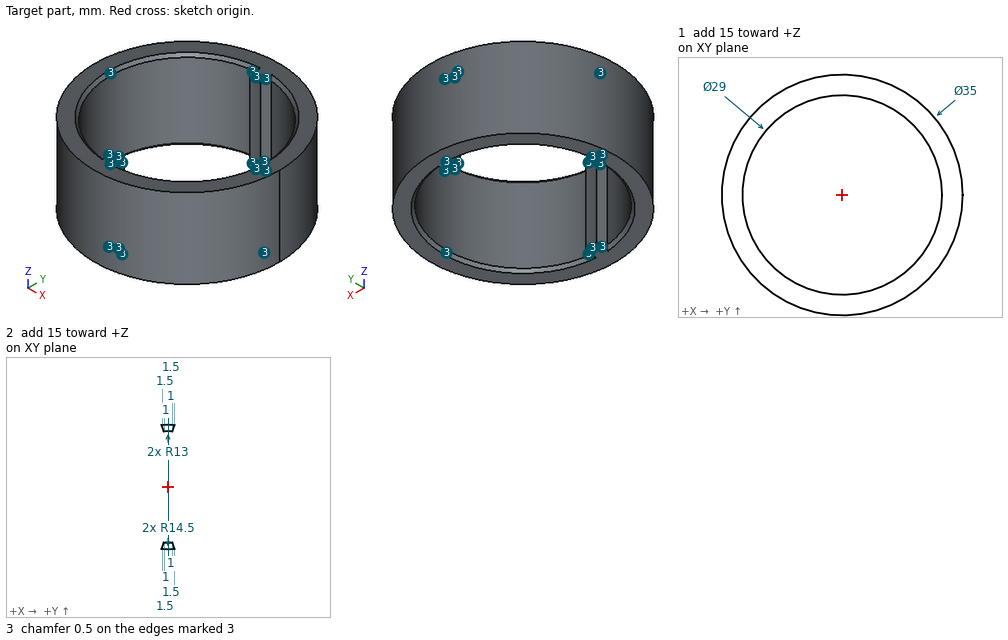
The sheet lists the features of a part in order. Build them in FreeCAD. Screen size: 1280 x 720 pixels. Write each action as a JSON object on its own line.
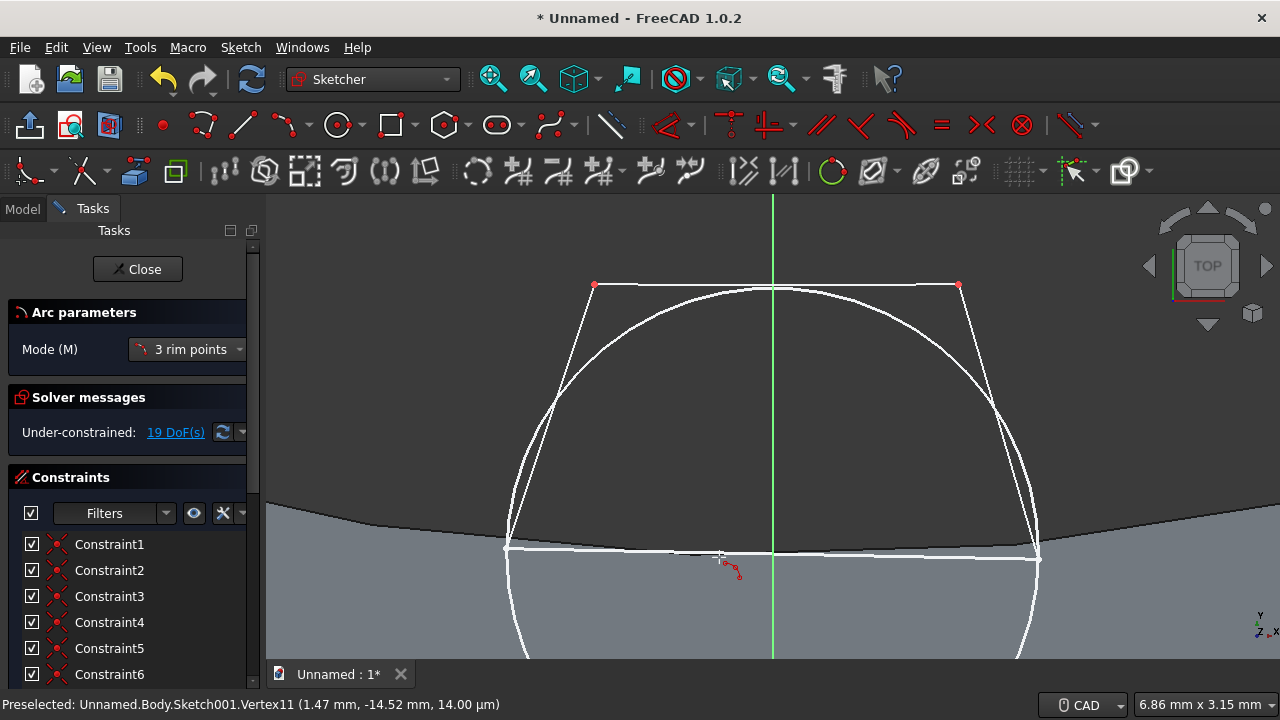
{"action": "left_click", "coordinate": [719, 555]}
{"action": "key", "text": "Escape"}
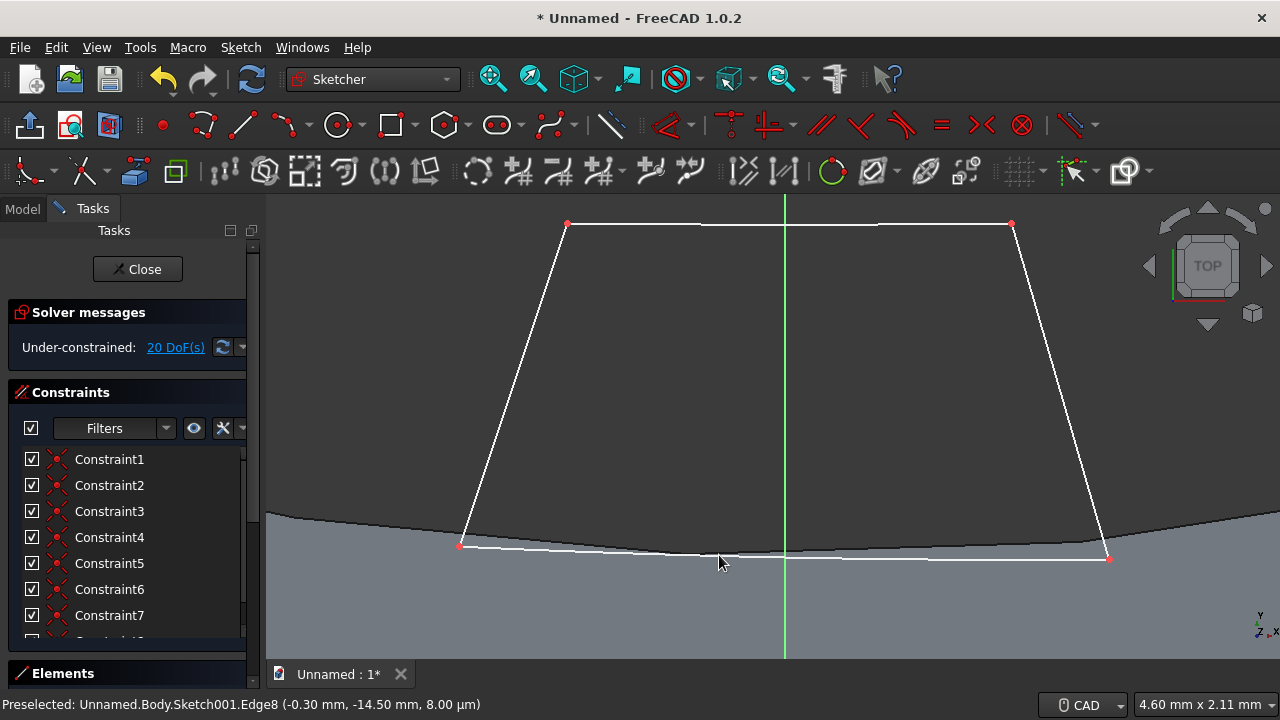
{"action": "scroll", "coordinate": [700, 587], "scroll_direction": "down", "scroll_amount": 15}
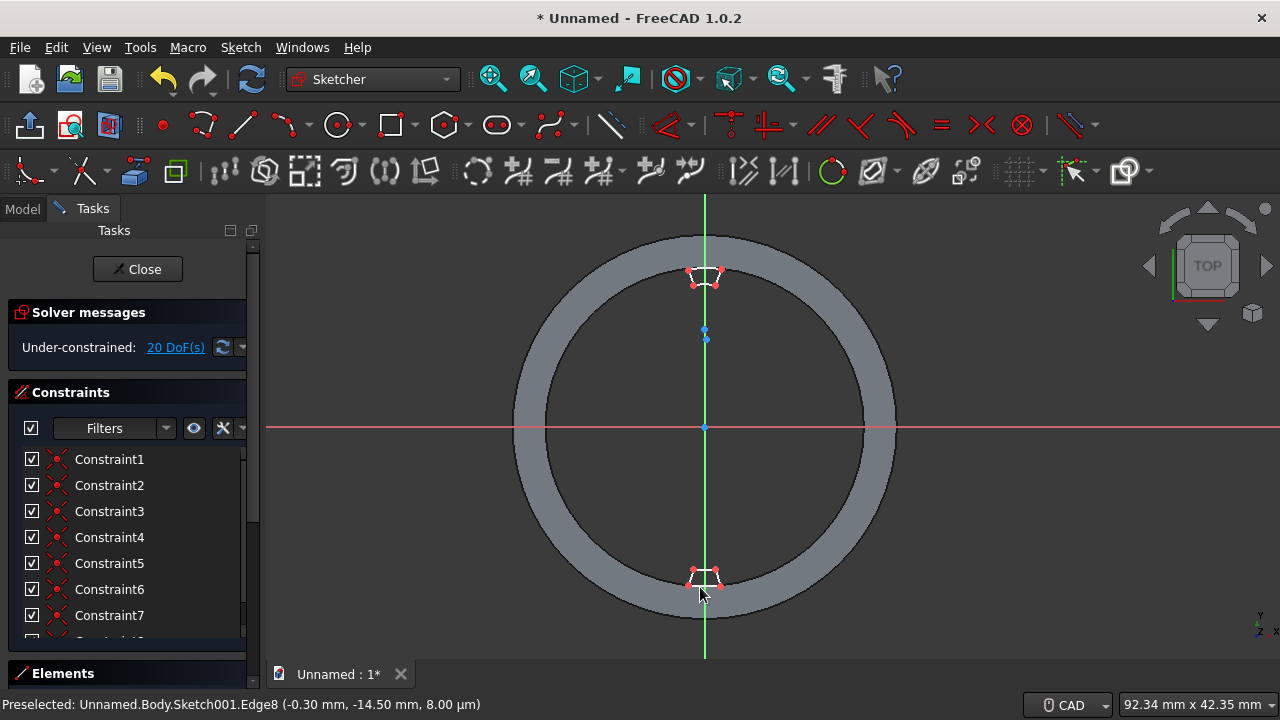
{"action": "scroll", "coordinate": [709, 284], "scroll_direction": "up", "scroll_amount": 6}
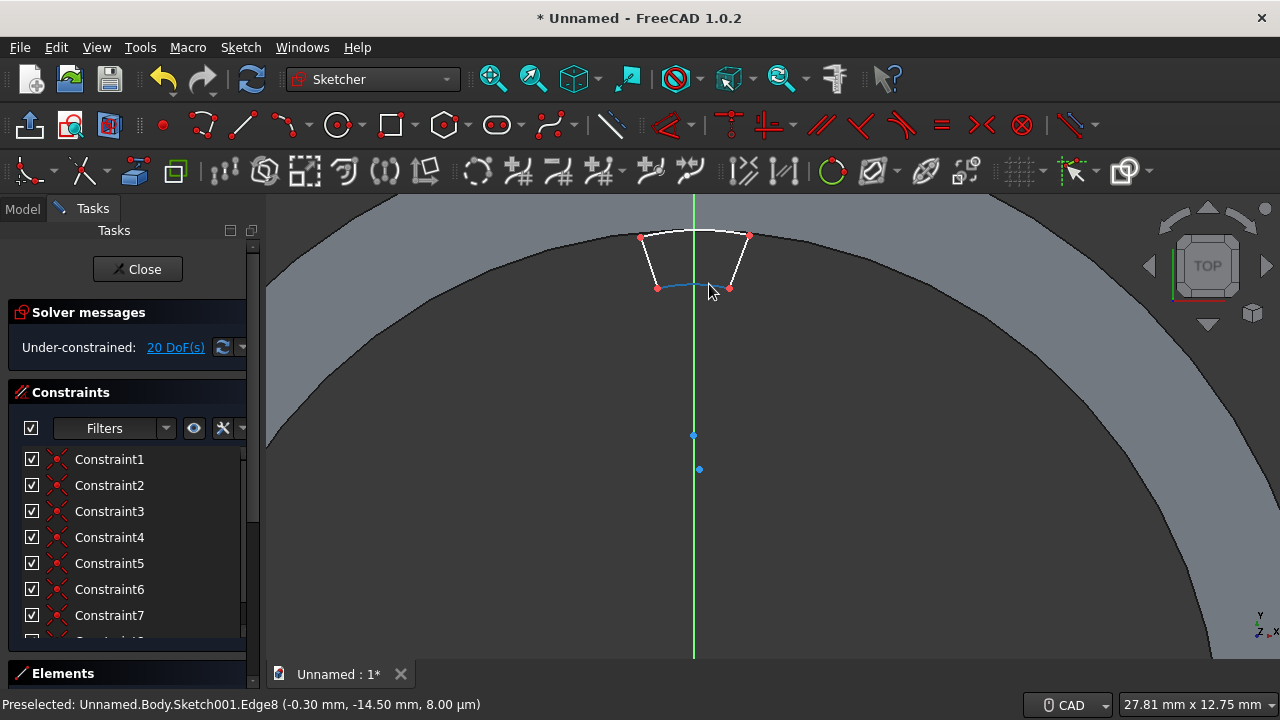
{"action": "left_click", "coordinate": [708, 285]}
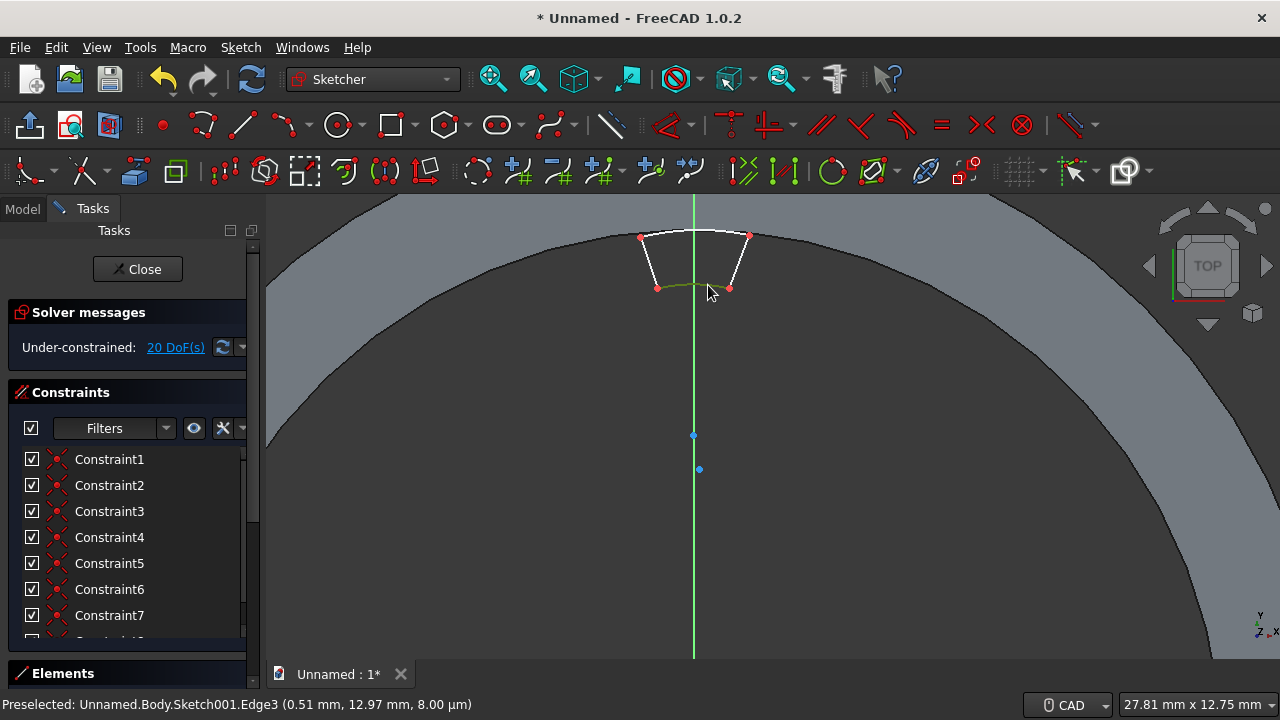
{"action": "left_click", "coordinate": [717, 231]}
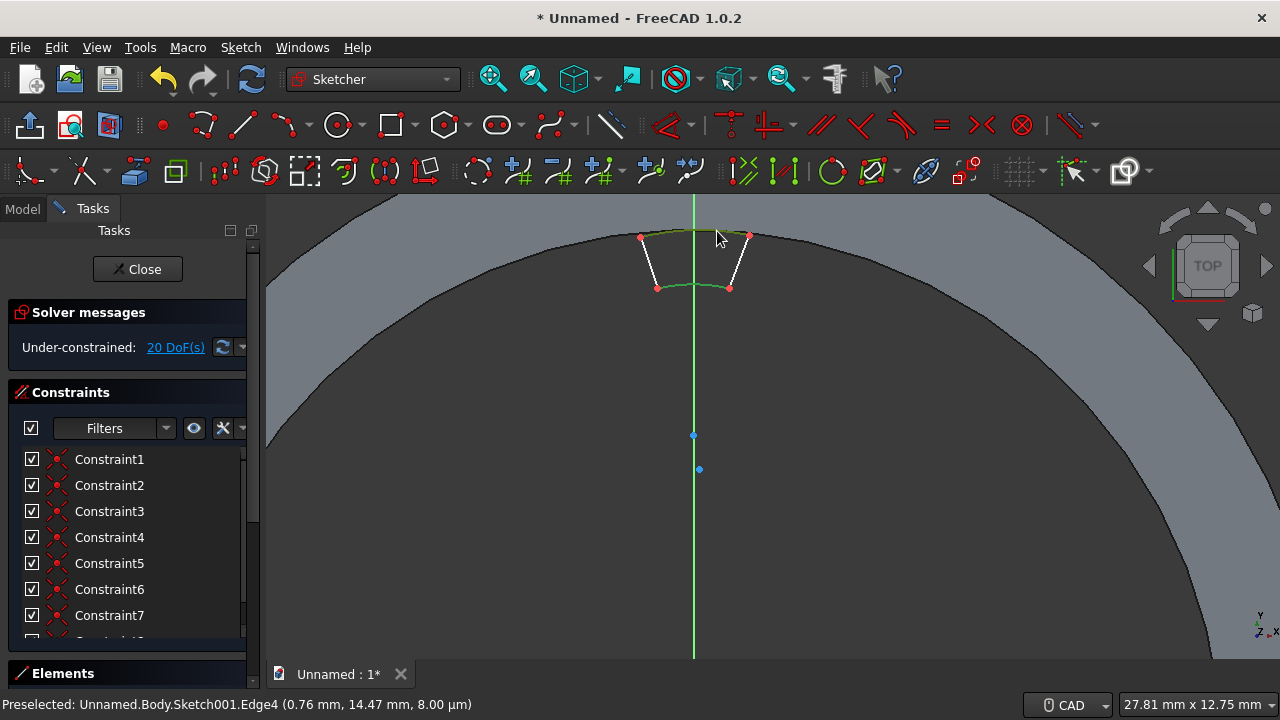
{"action": "left_click", "coordinate": [730, 126]}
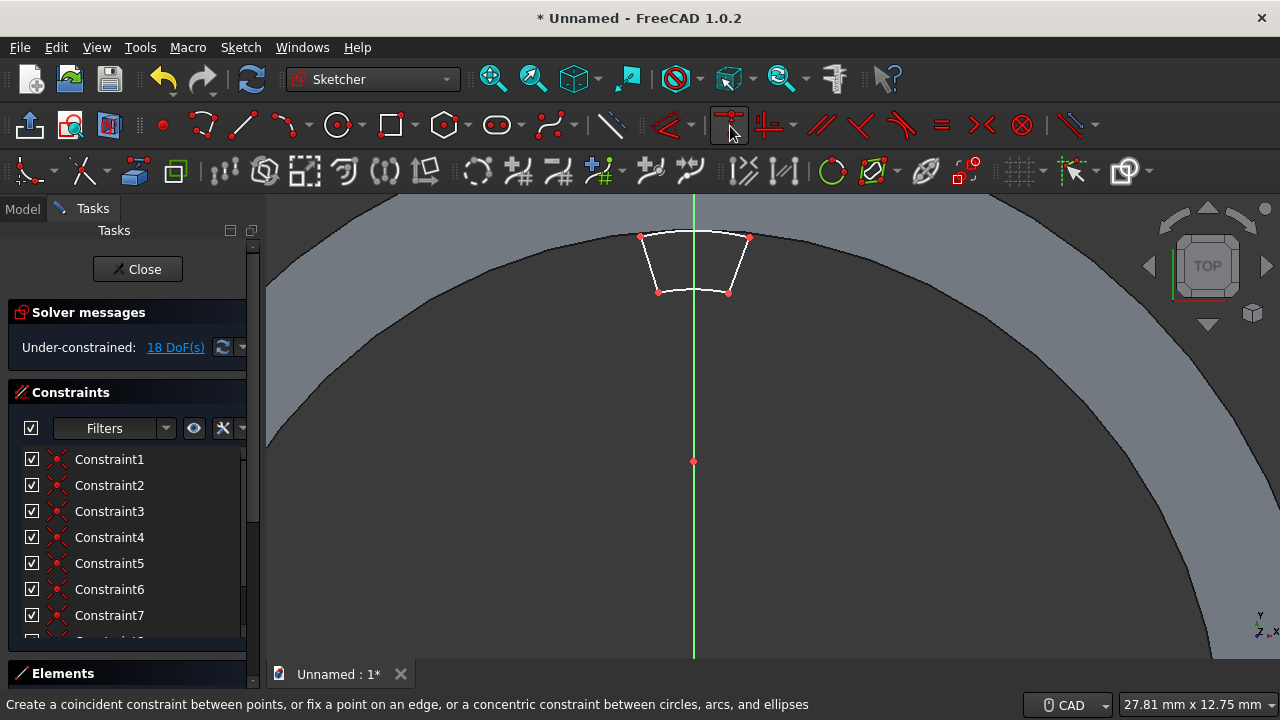
{"action": "left_click", "coordinate": [708, 290]}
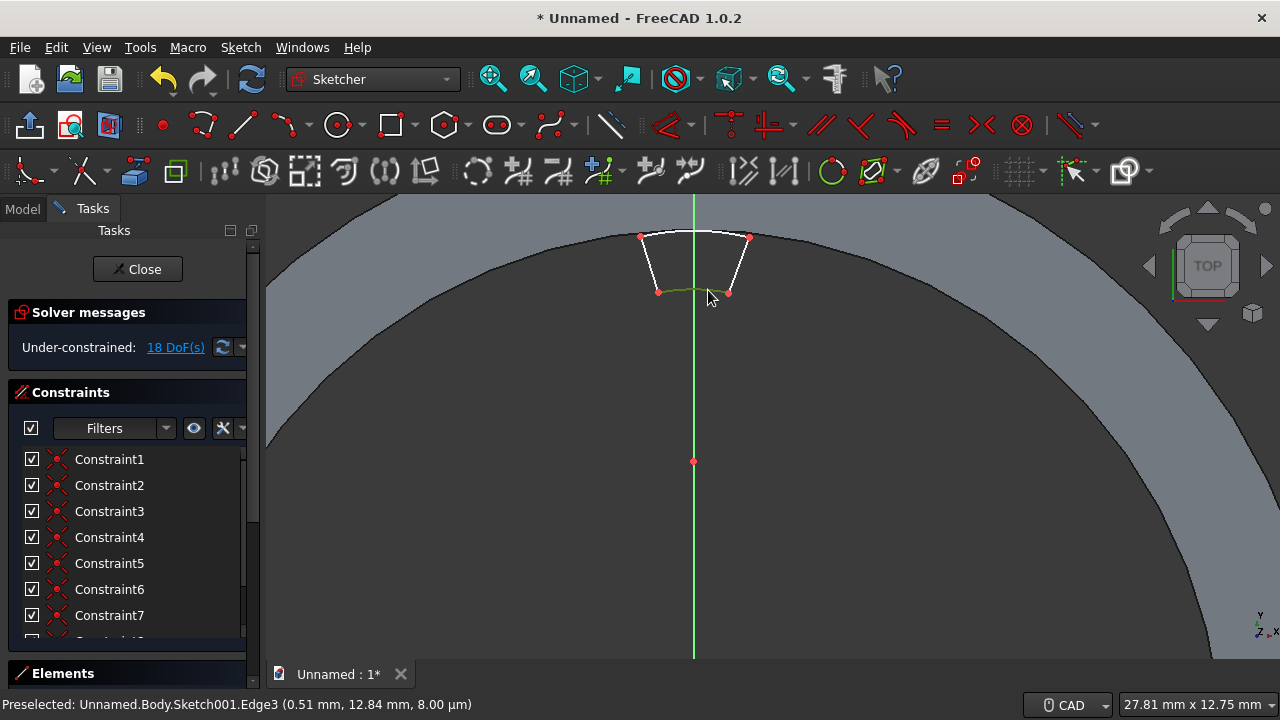
{"action": "scroll", "coordinate": [709, 283], "scroll_direction": "down", "scroll_amount": 6}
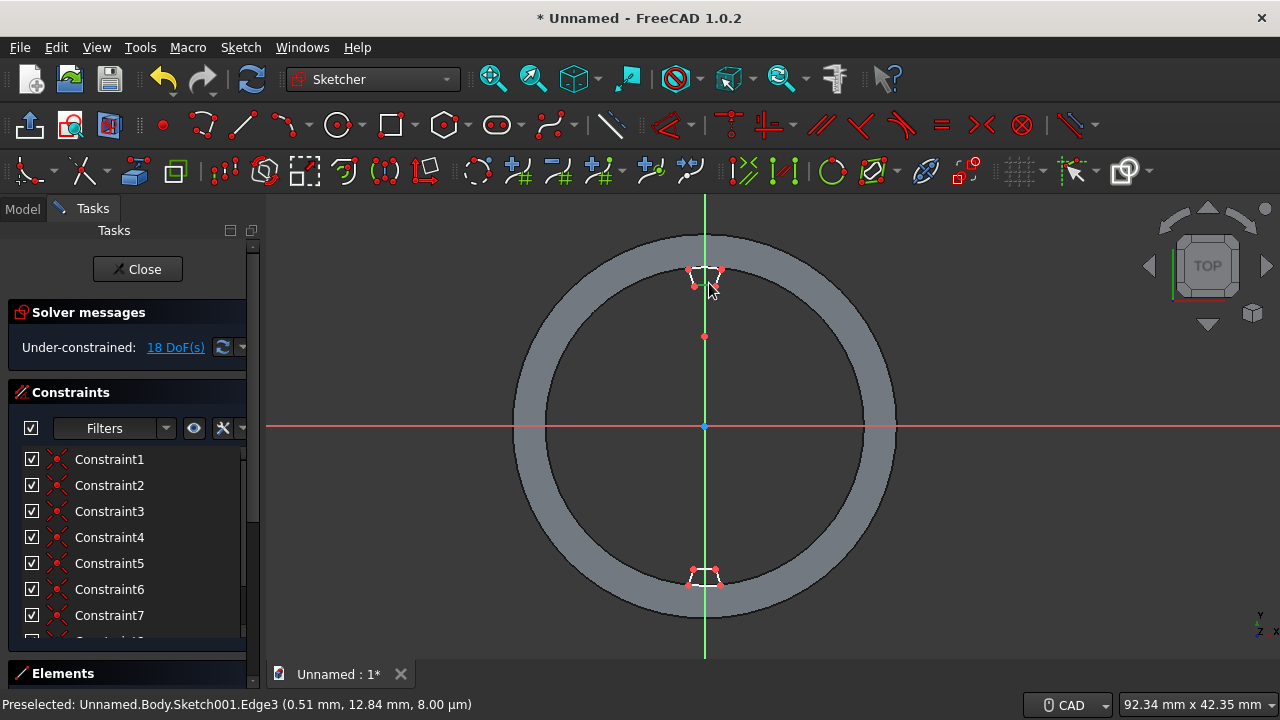
{"action": "scroll", "coordinate": [700, 569], "scroll_direction": "up", "scroll_amount": 6}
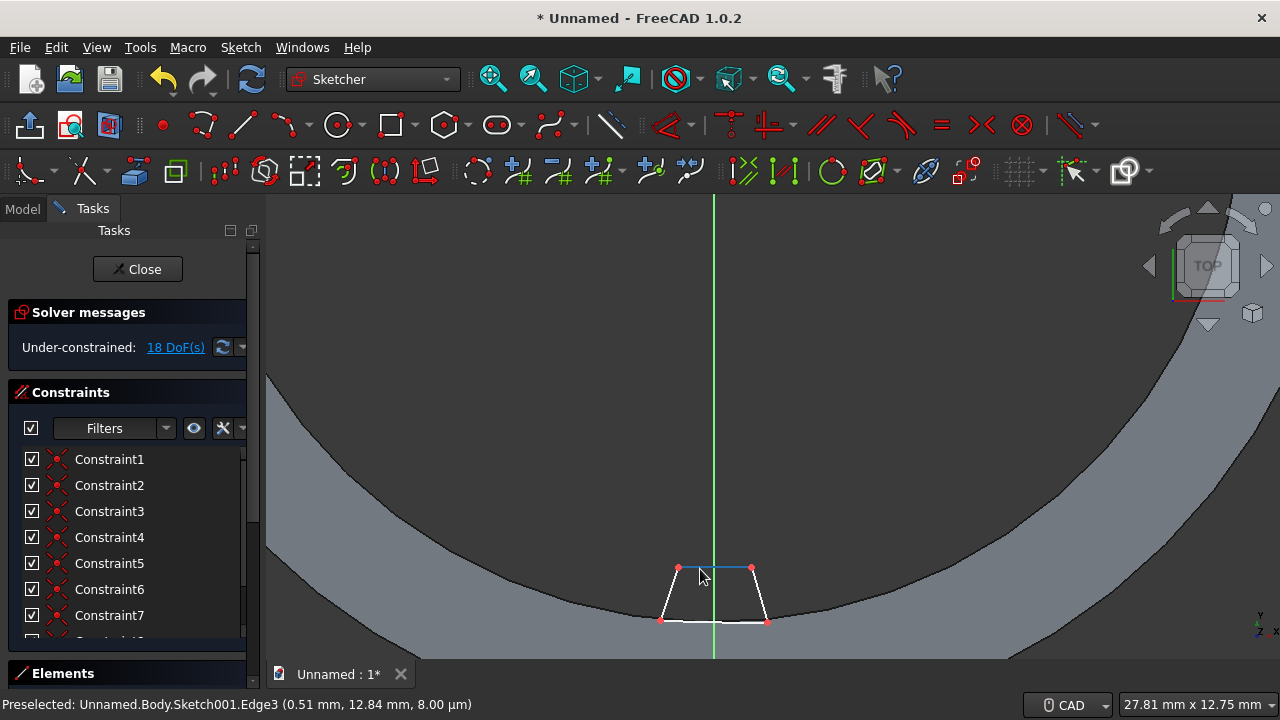
{"action": "left_click", "coordinate": [700, 567]}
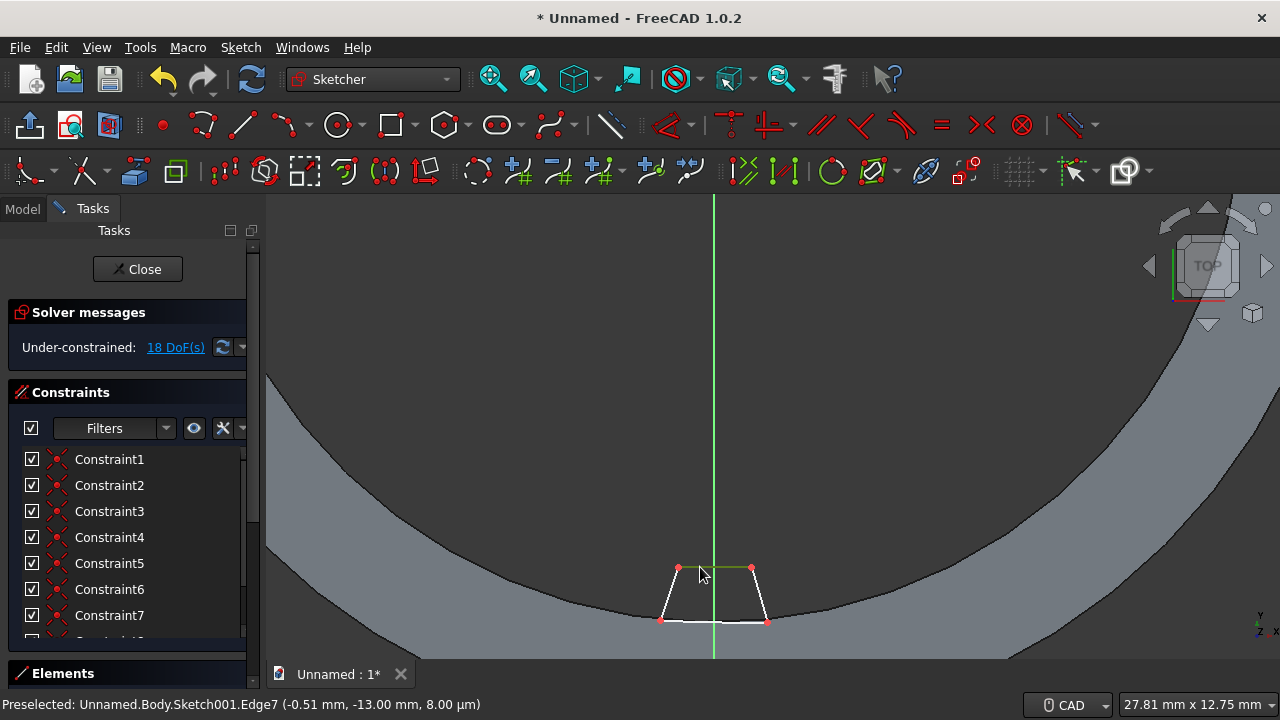
{"action": "left_click", "coordinate": [730, 126]}